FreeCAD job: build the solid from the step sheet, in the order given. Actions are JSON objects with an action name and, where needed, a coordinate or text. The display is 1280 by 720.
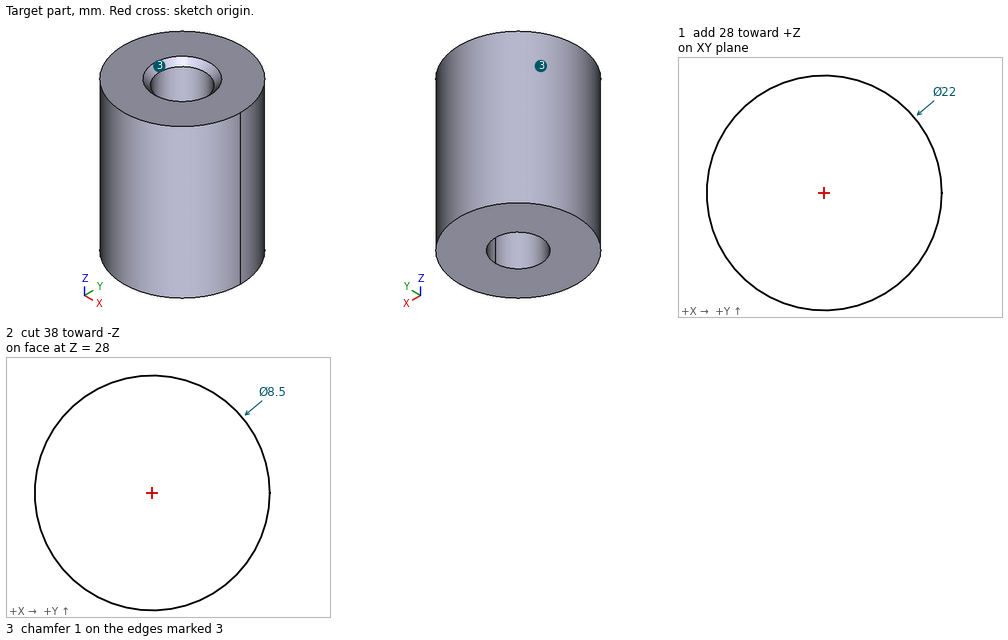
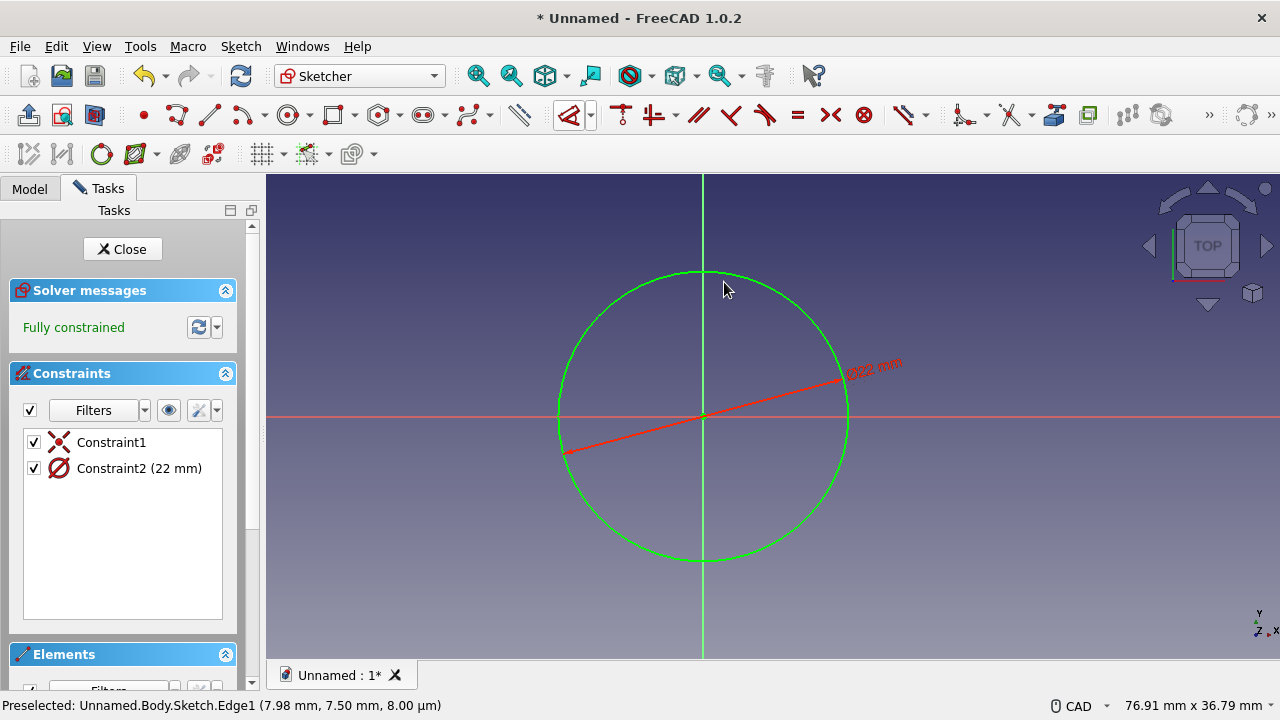
{"action": "left_click", "coordinate": [123, 249]}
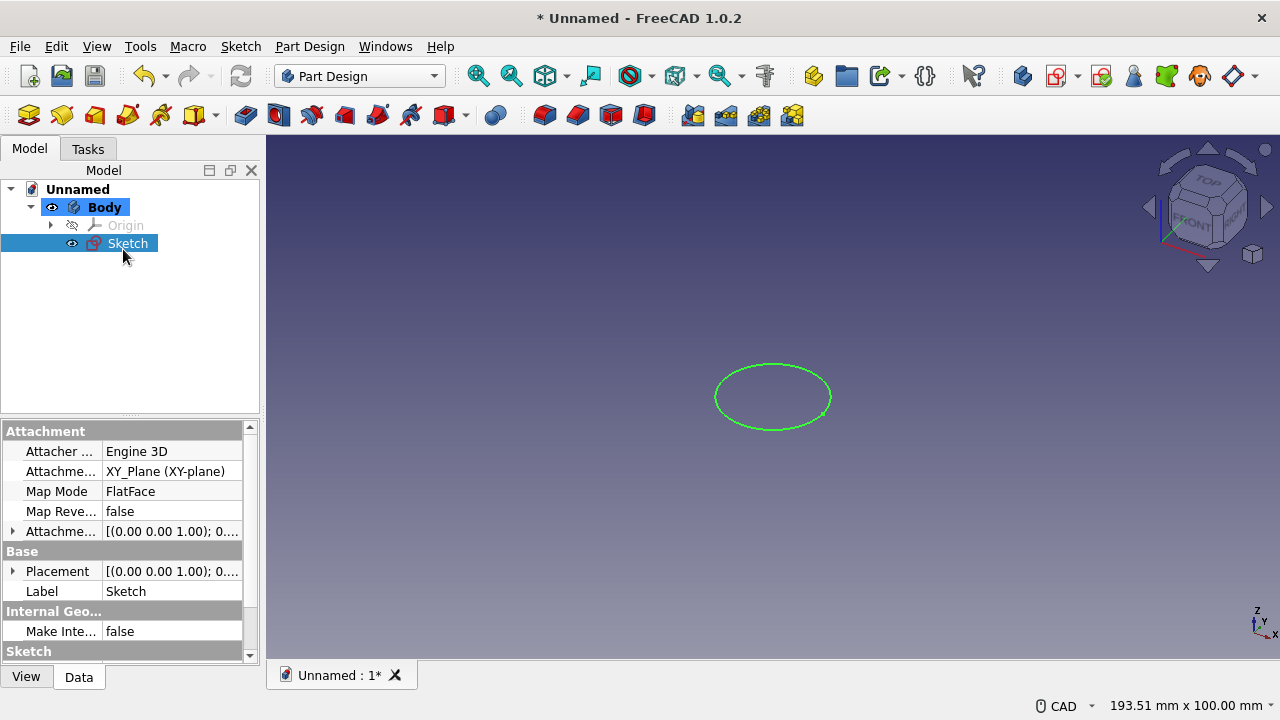
{"action": "left_click", "coordinate": [29, 116]}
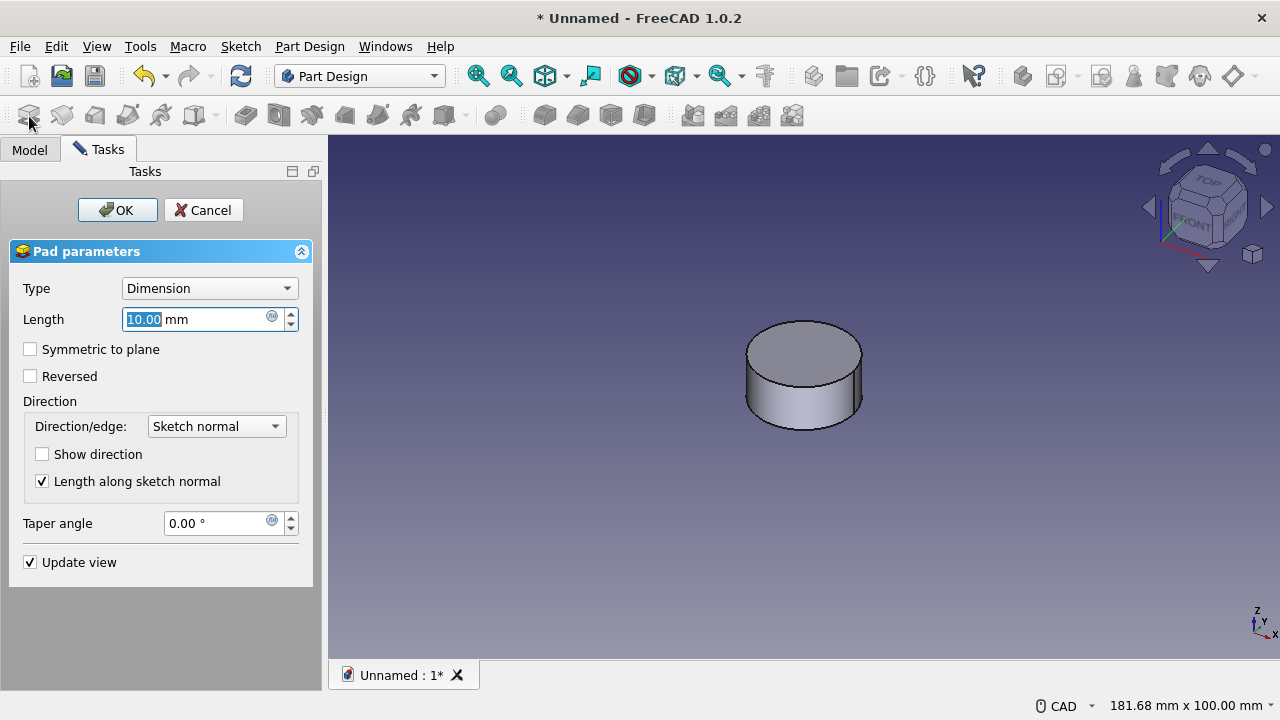
{"action": "type", "text": "28"}
{"action": "key", "text": "Tab"}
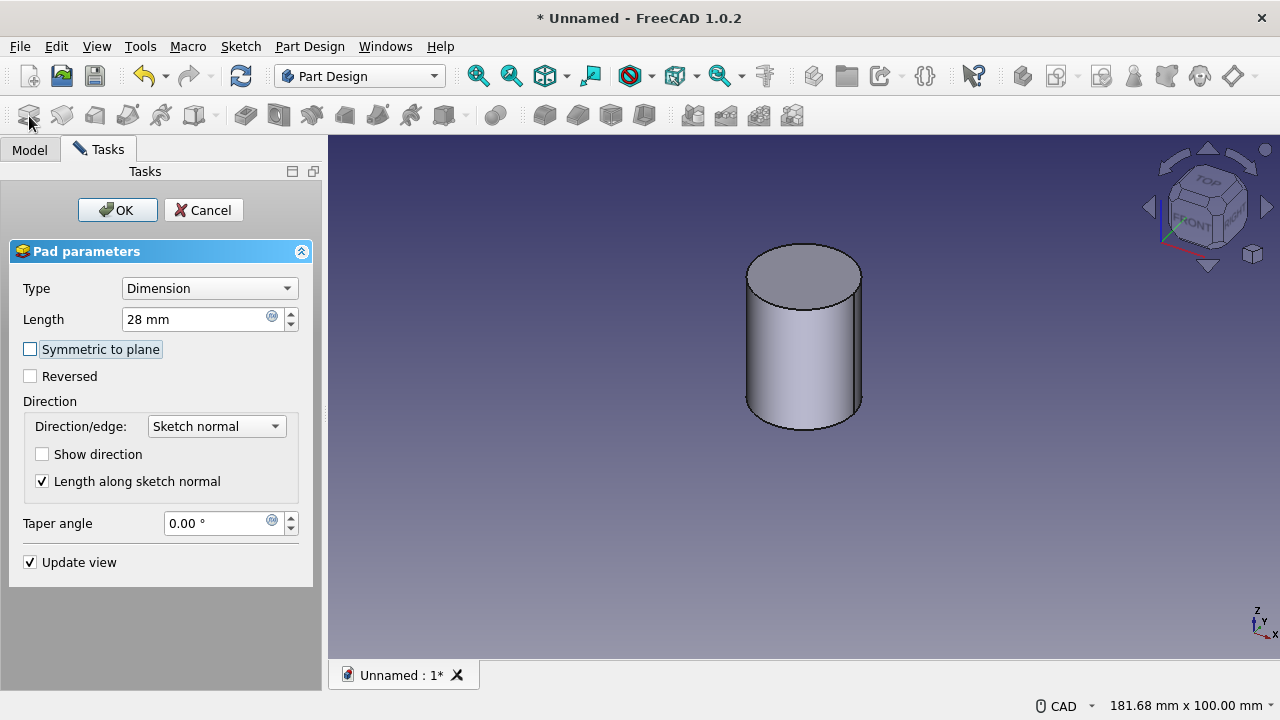
{"action": "left_click", "coordinate": [118, 210]}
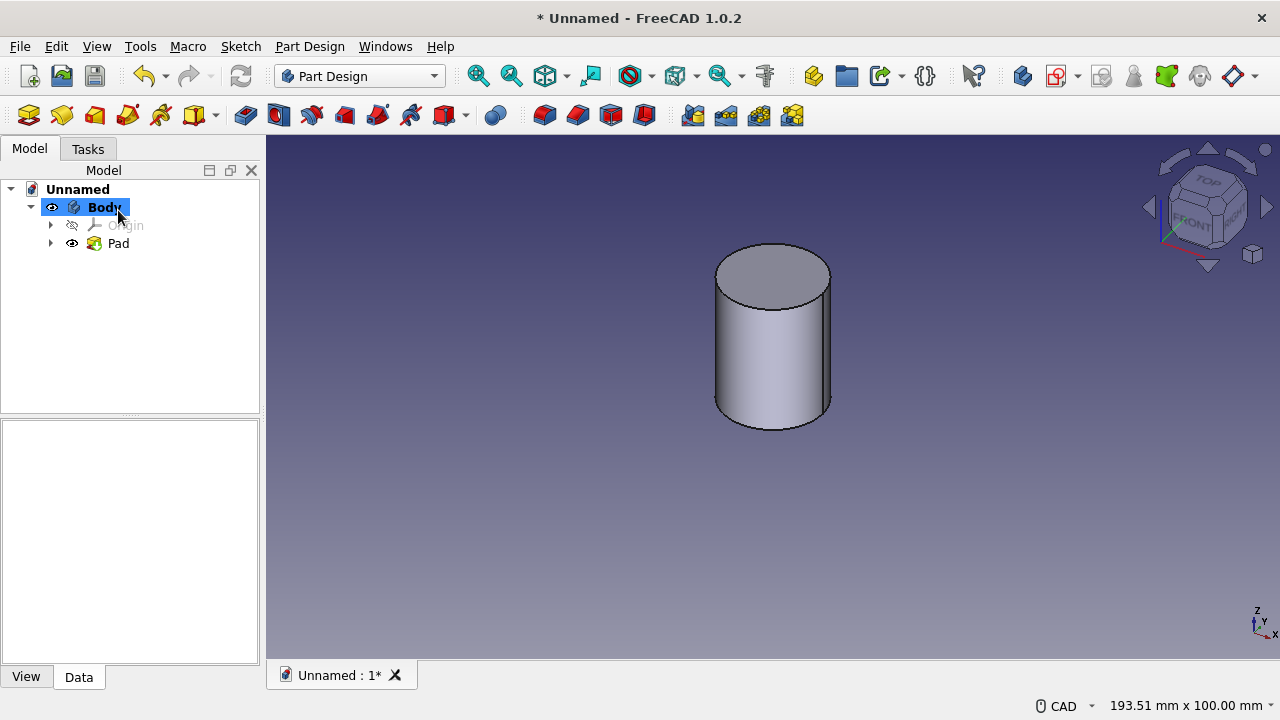
{"action": "left_click", "coordinate": [479, 76]}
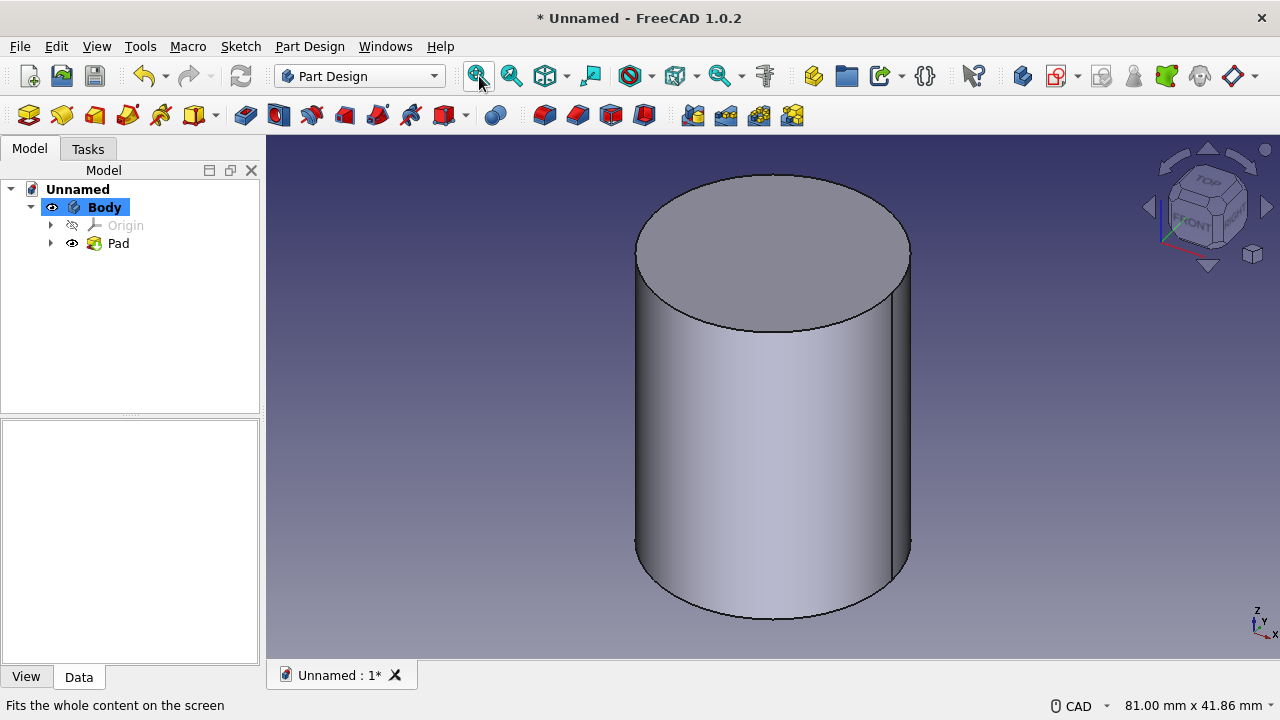
{"action": "left_click", "coordinate": [773, 252]}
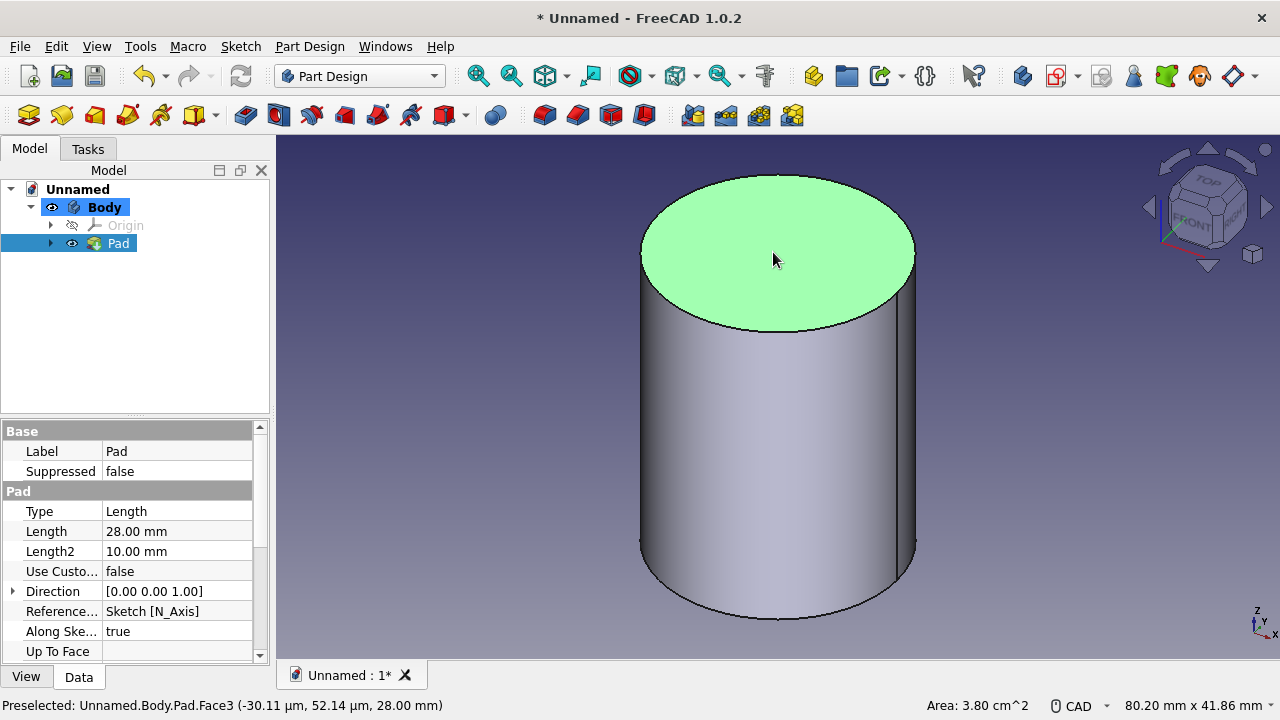
{"action": "left_click", "coordinate": [1056, 76]}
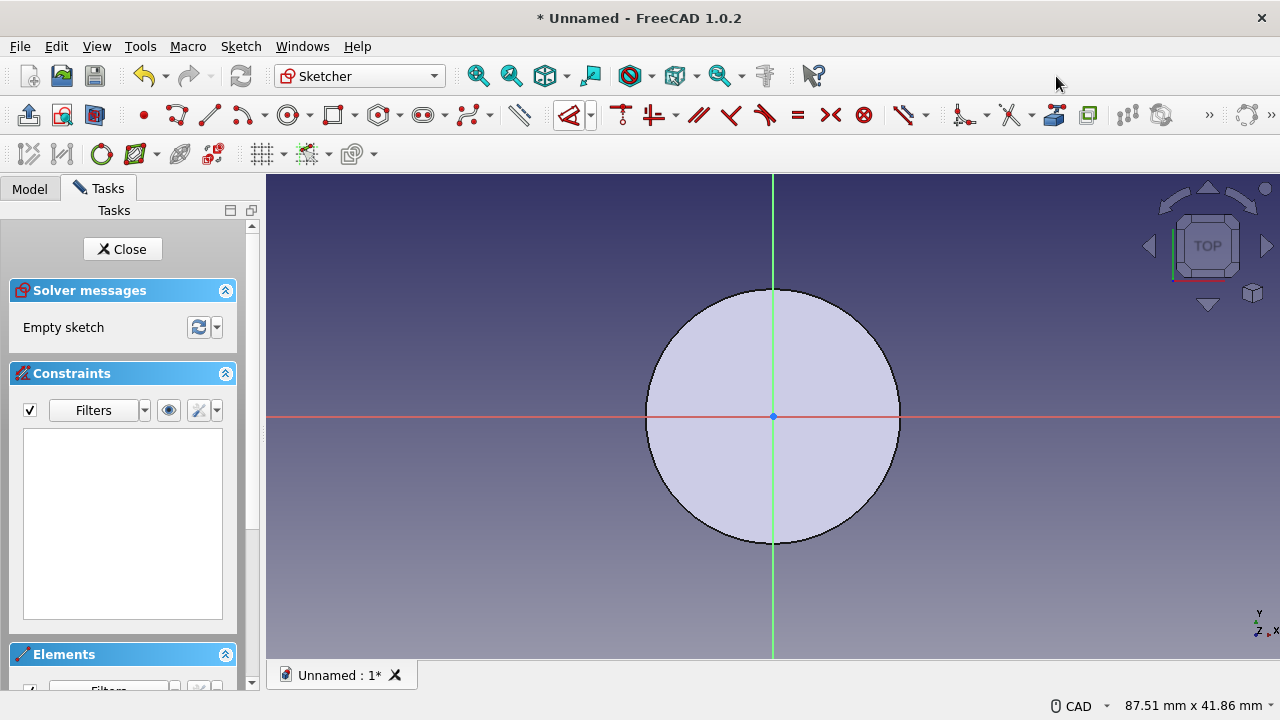
{"action": "scroll", "coordinate": [803, 416], "scroll_direction": "up", "scroll_amount": 6}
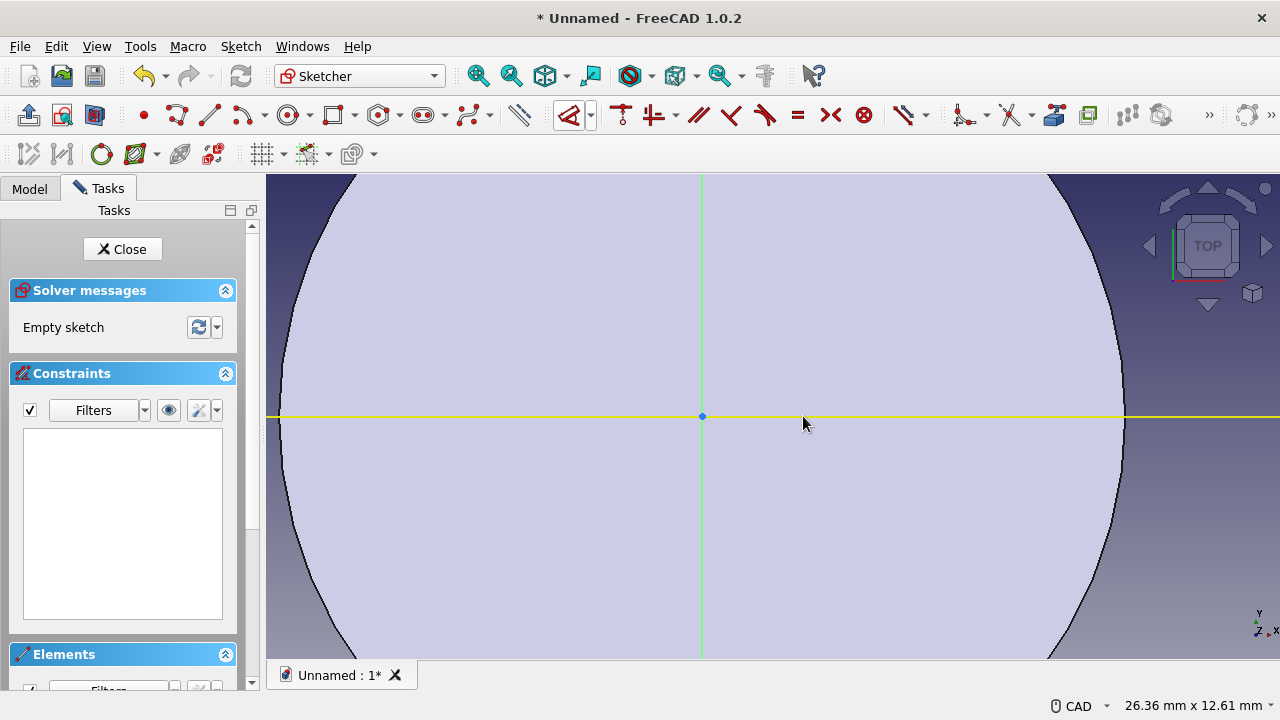
{"action": "key", "text": "g c"}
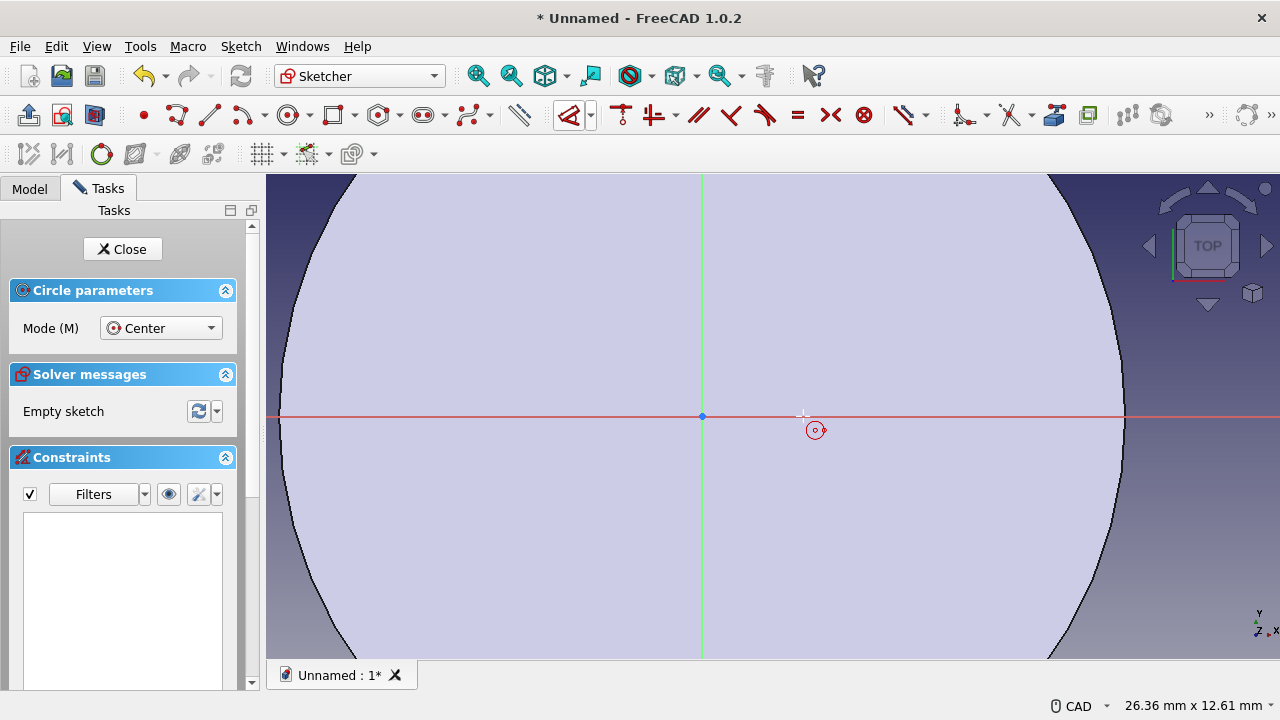
{"action": "left_click", "coordinate": [702, 416]}
{"action": "left_click", "coordinate": [818, 301]}
{"action": "key", "text": "Escape"}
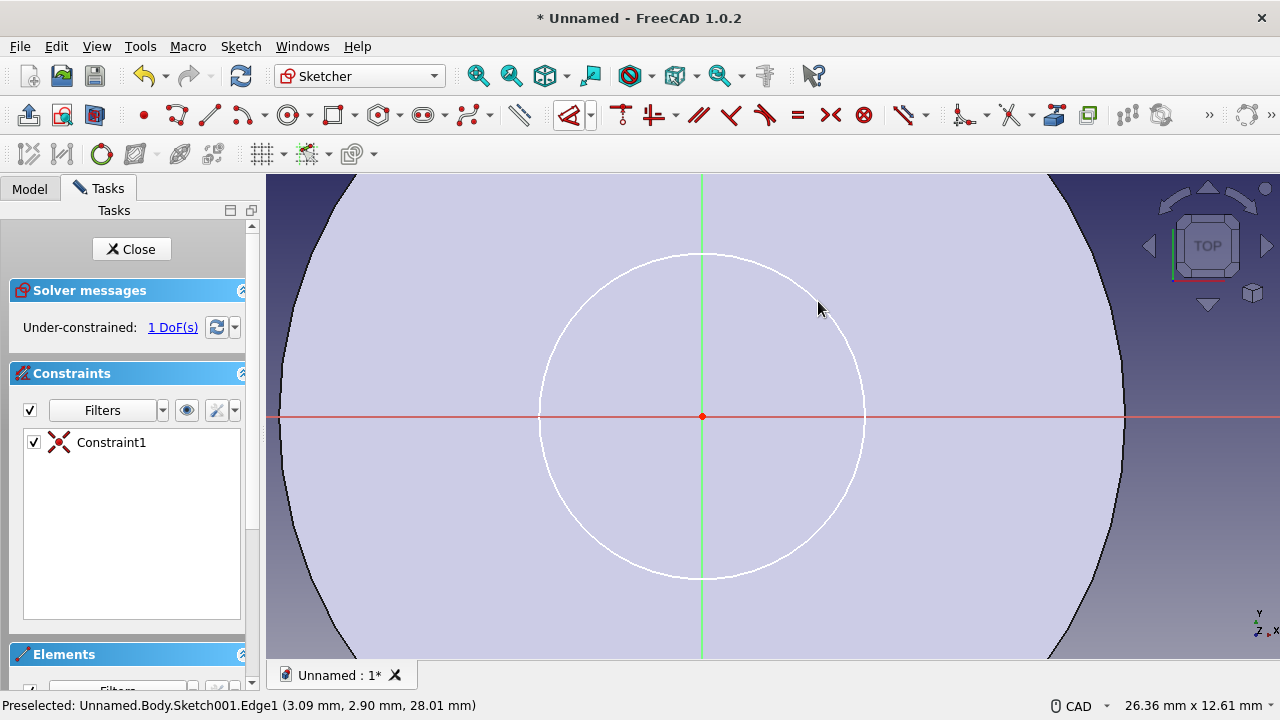
{"action": "left_click", "coordinate": [817, 301]}